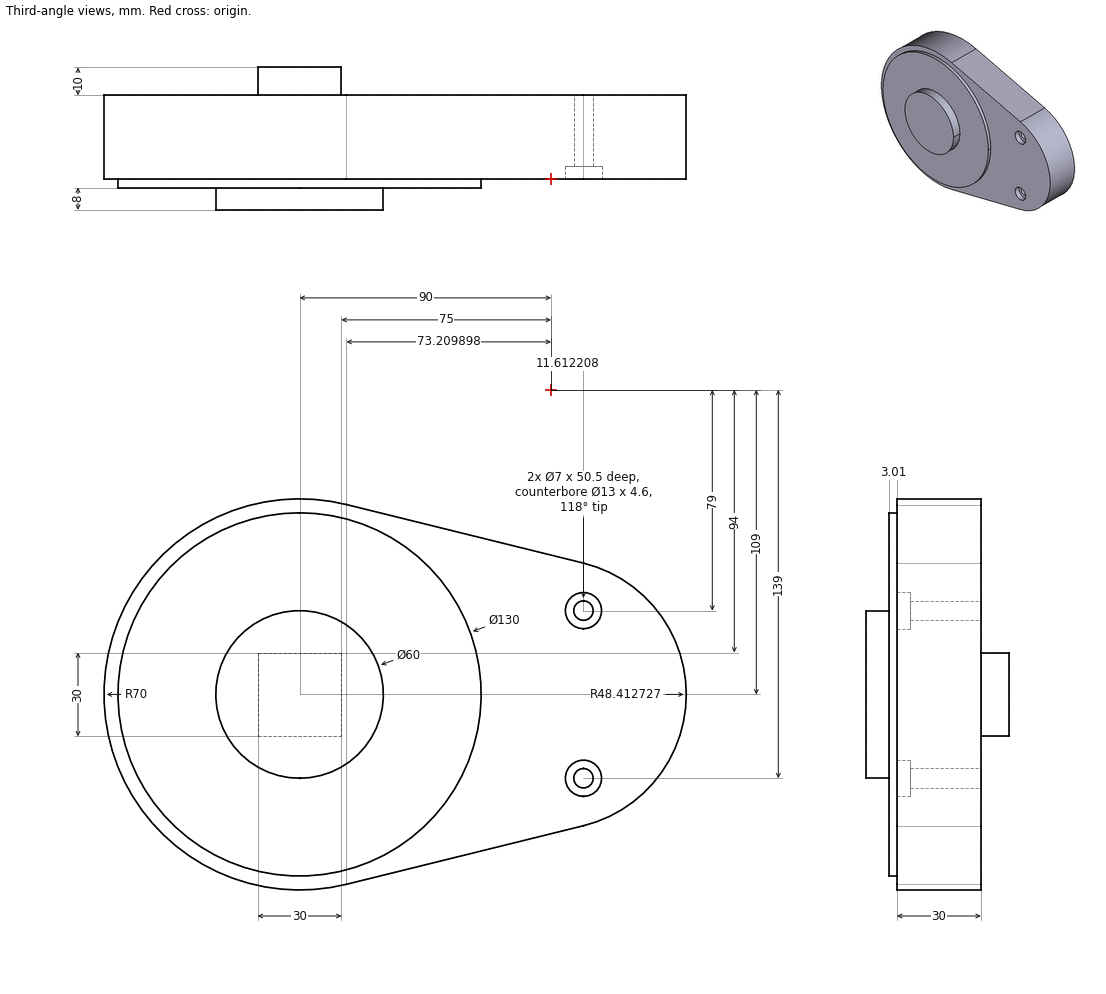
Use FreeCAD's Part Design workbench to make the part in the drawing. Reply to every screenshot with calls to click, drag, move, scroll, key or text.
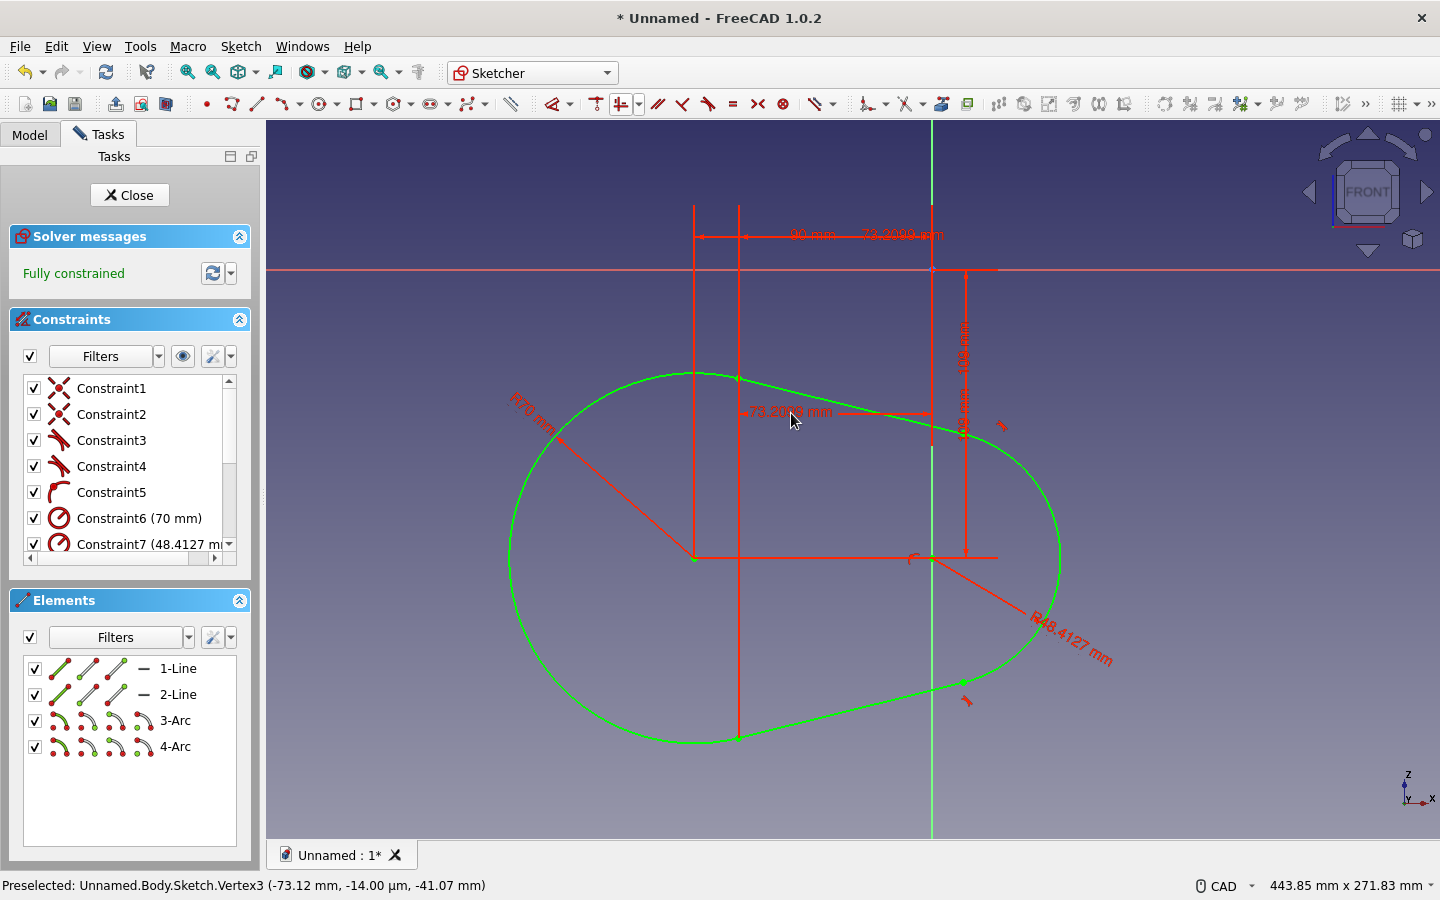
click(130, 195)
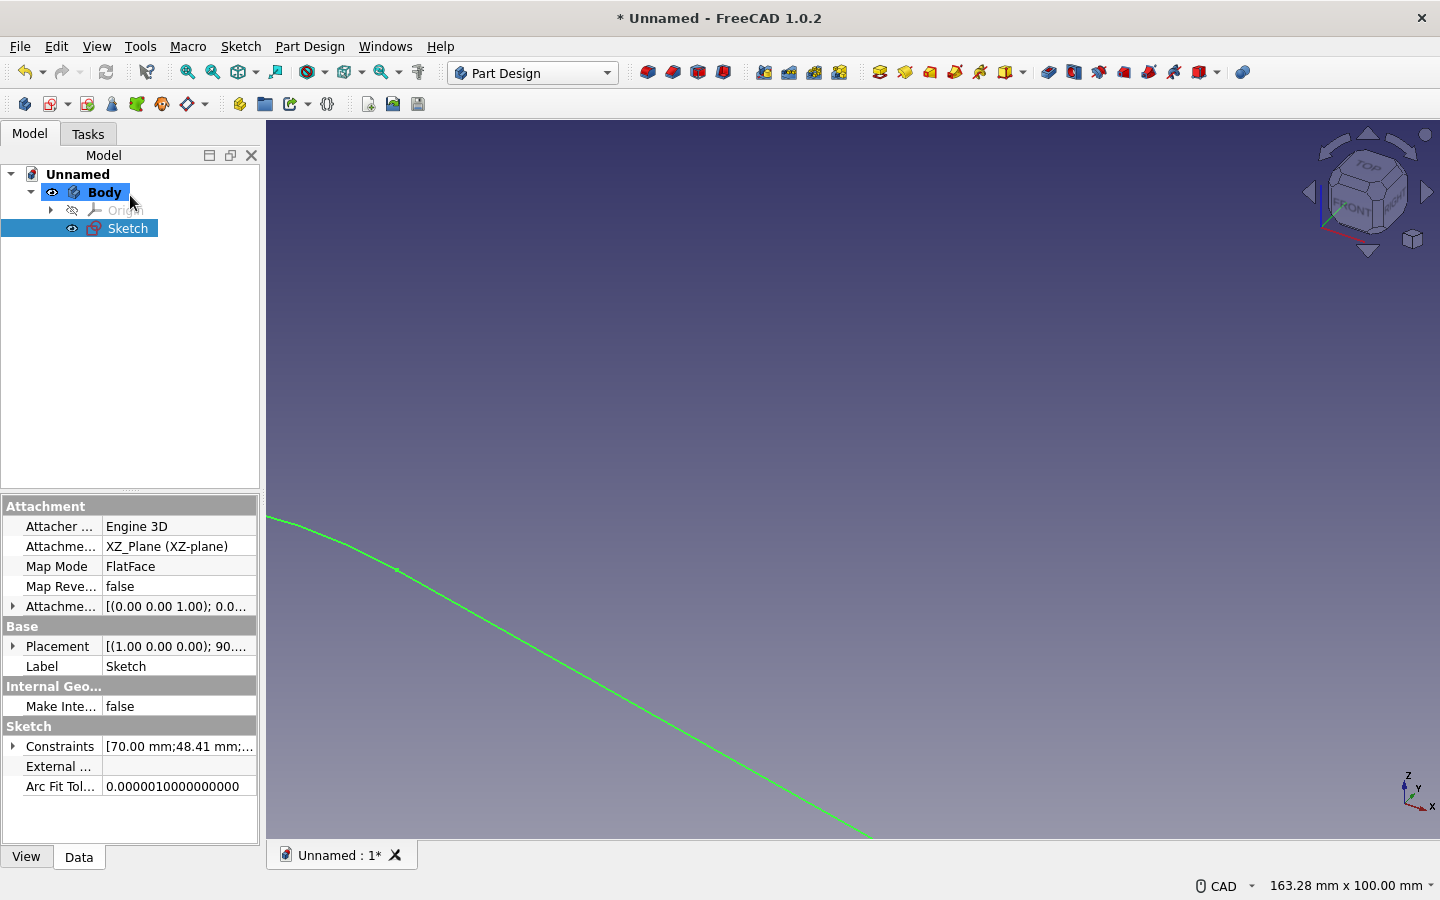
click(880, 72)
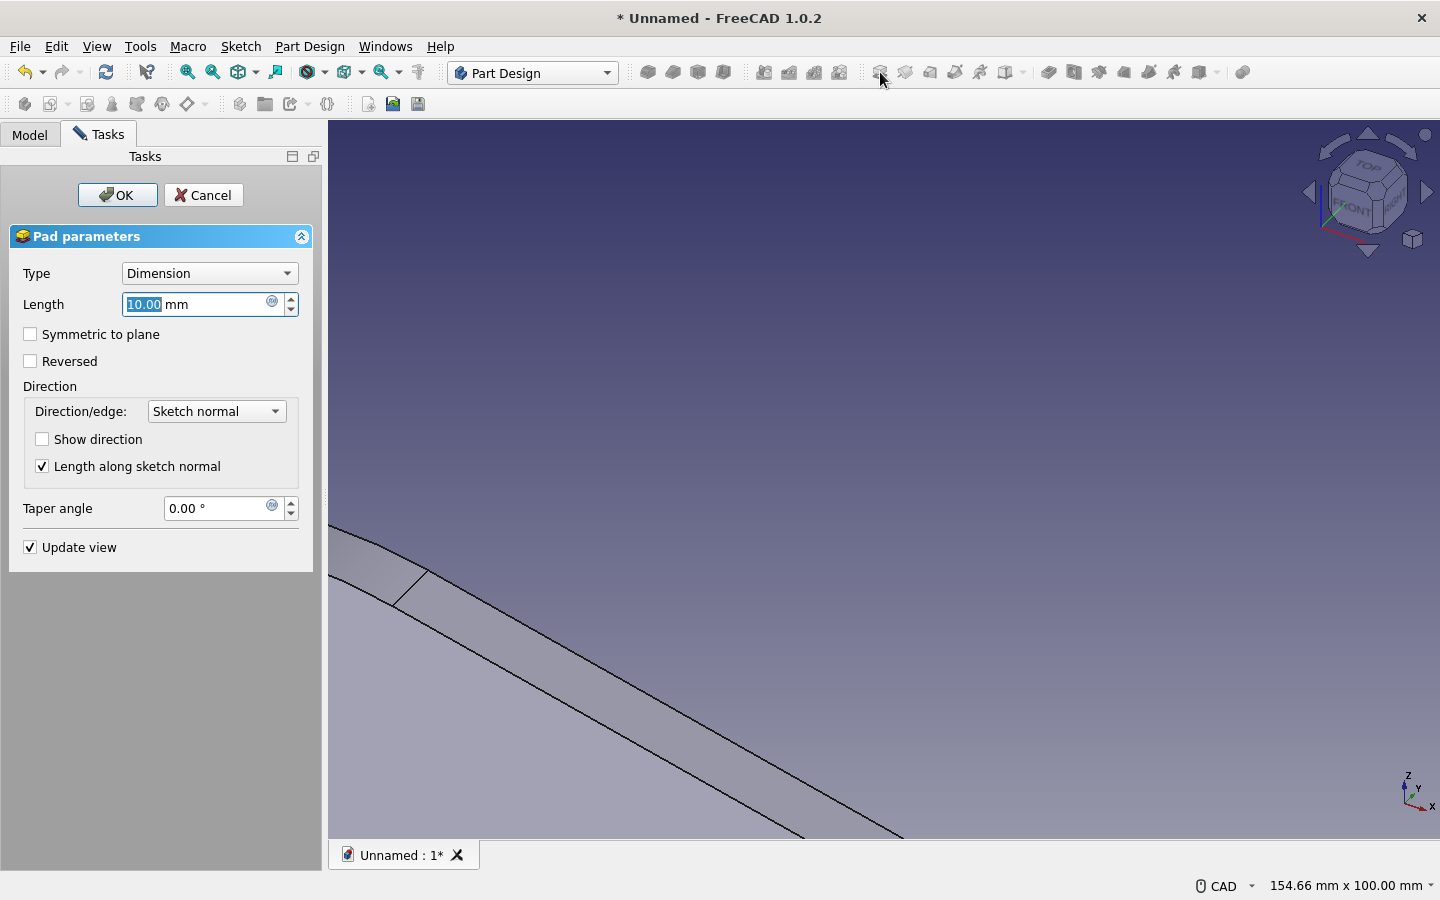
text(30)
key(Tab)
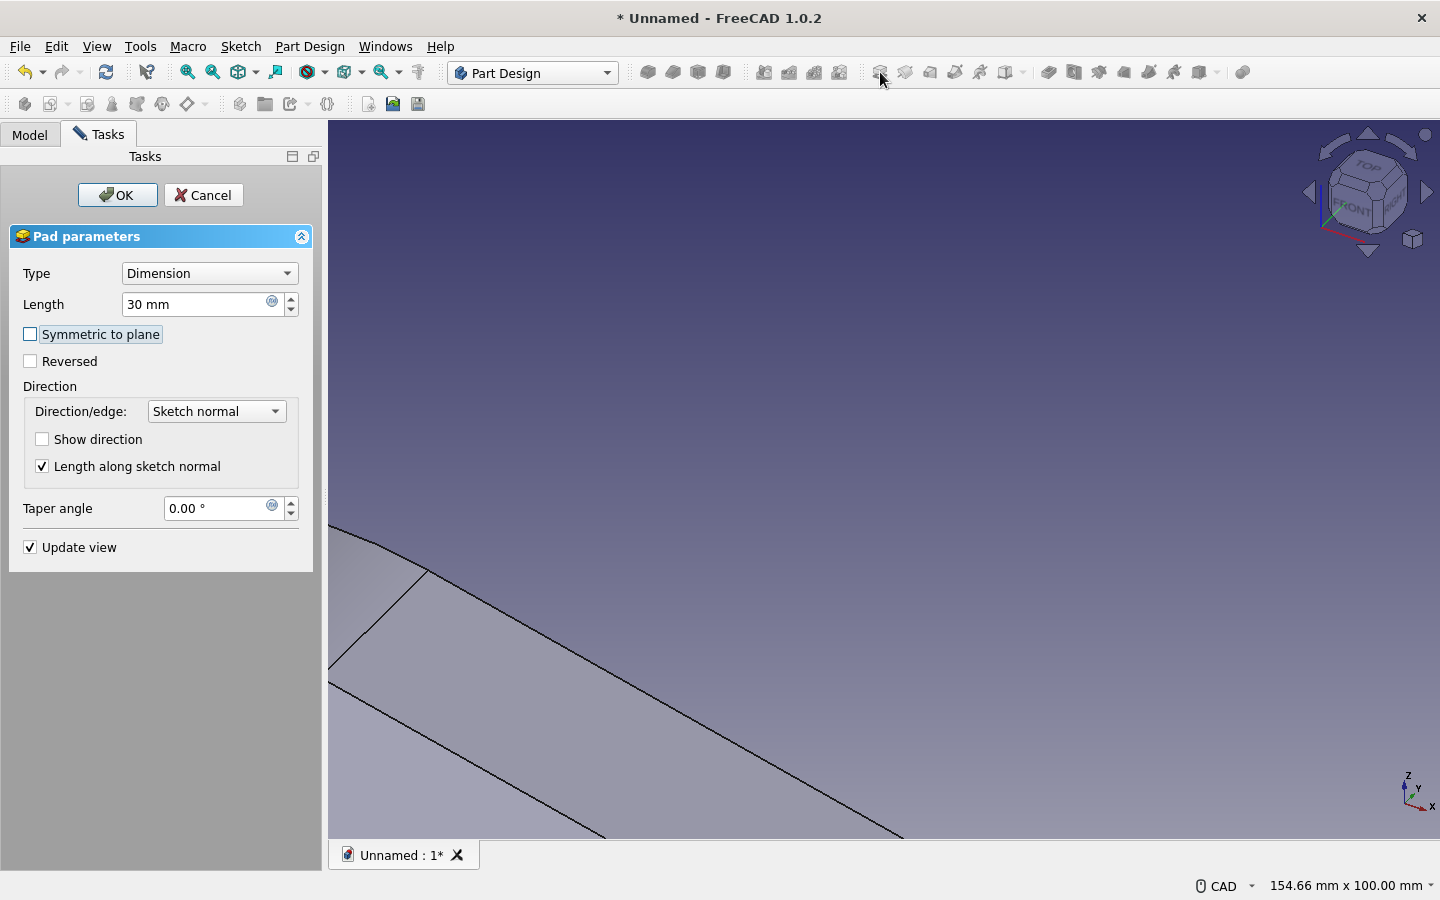
click(31, 361)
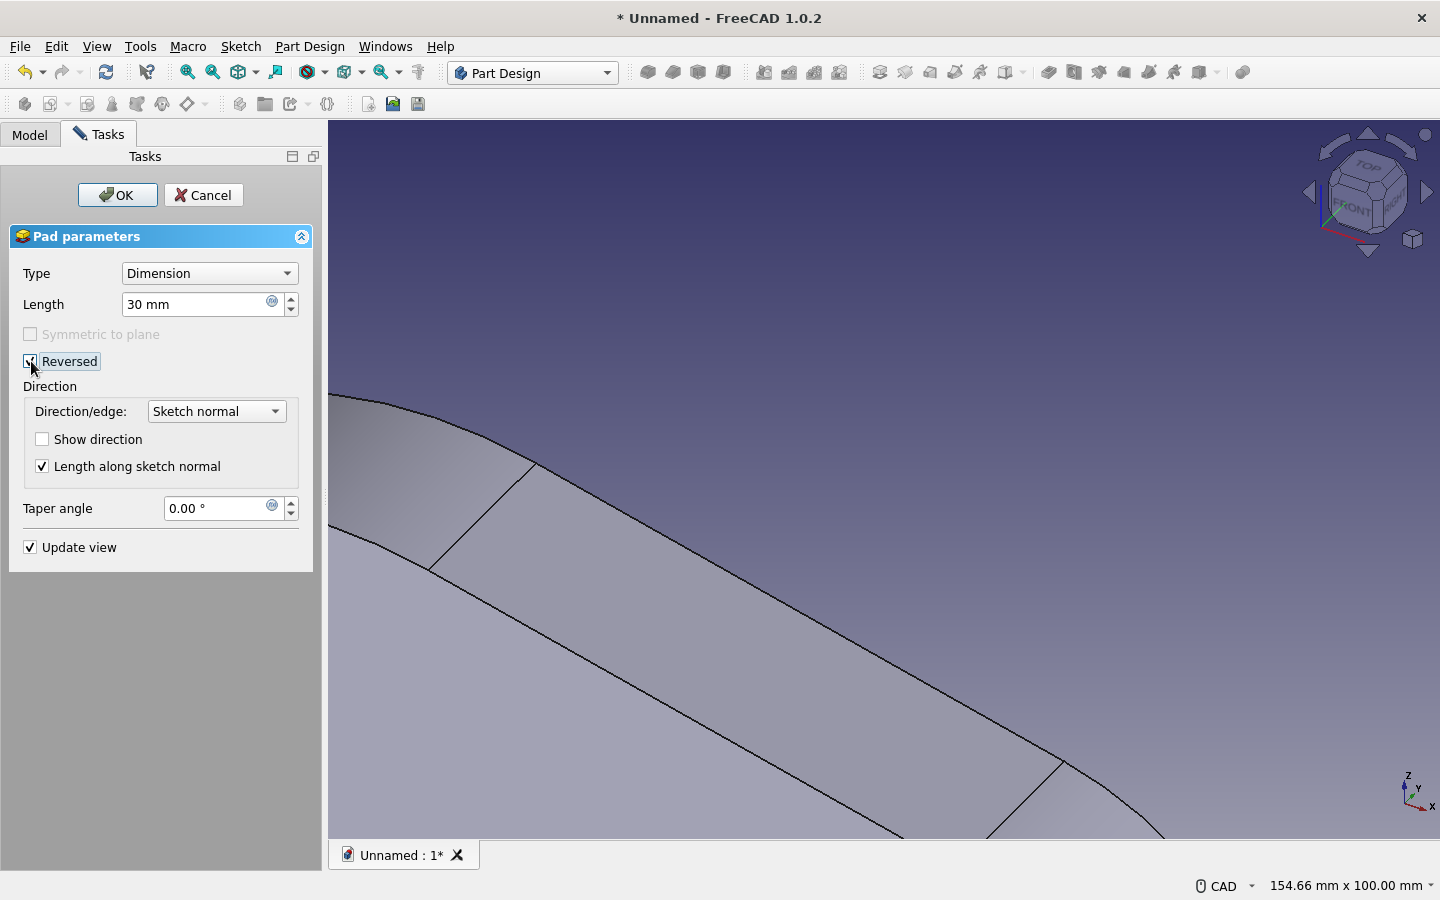
click(118, 195)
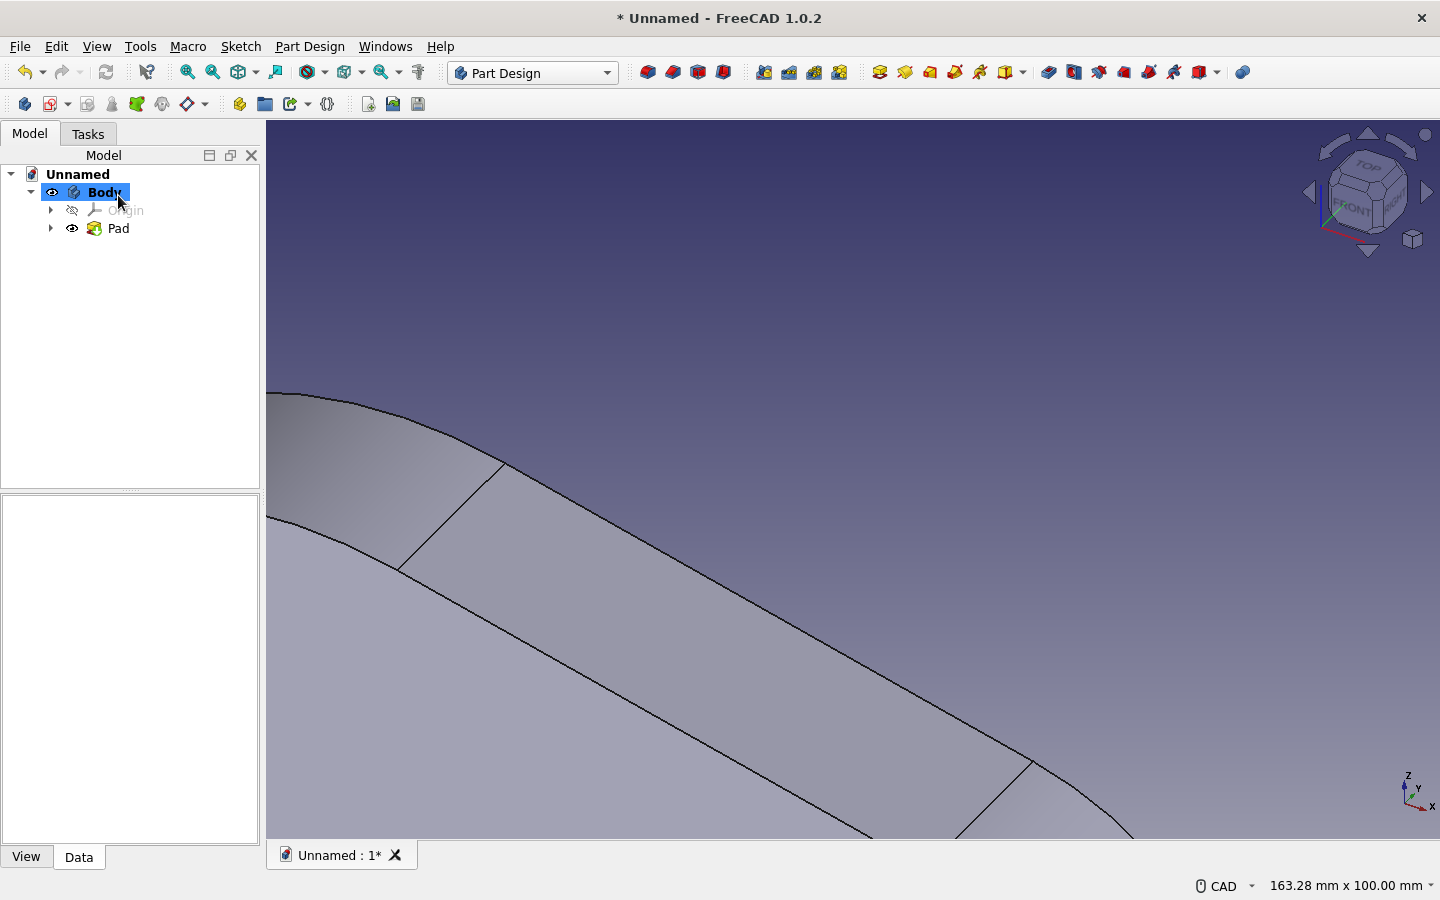
key(v)
key(f)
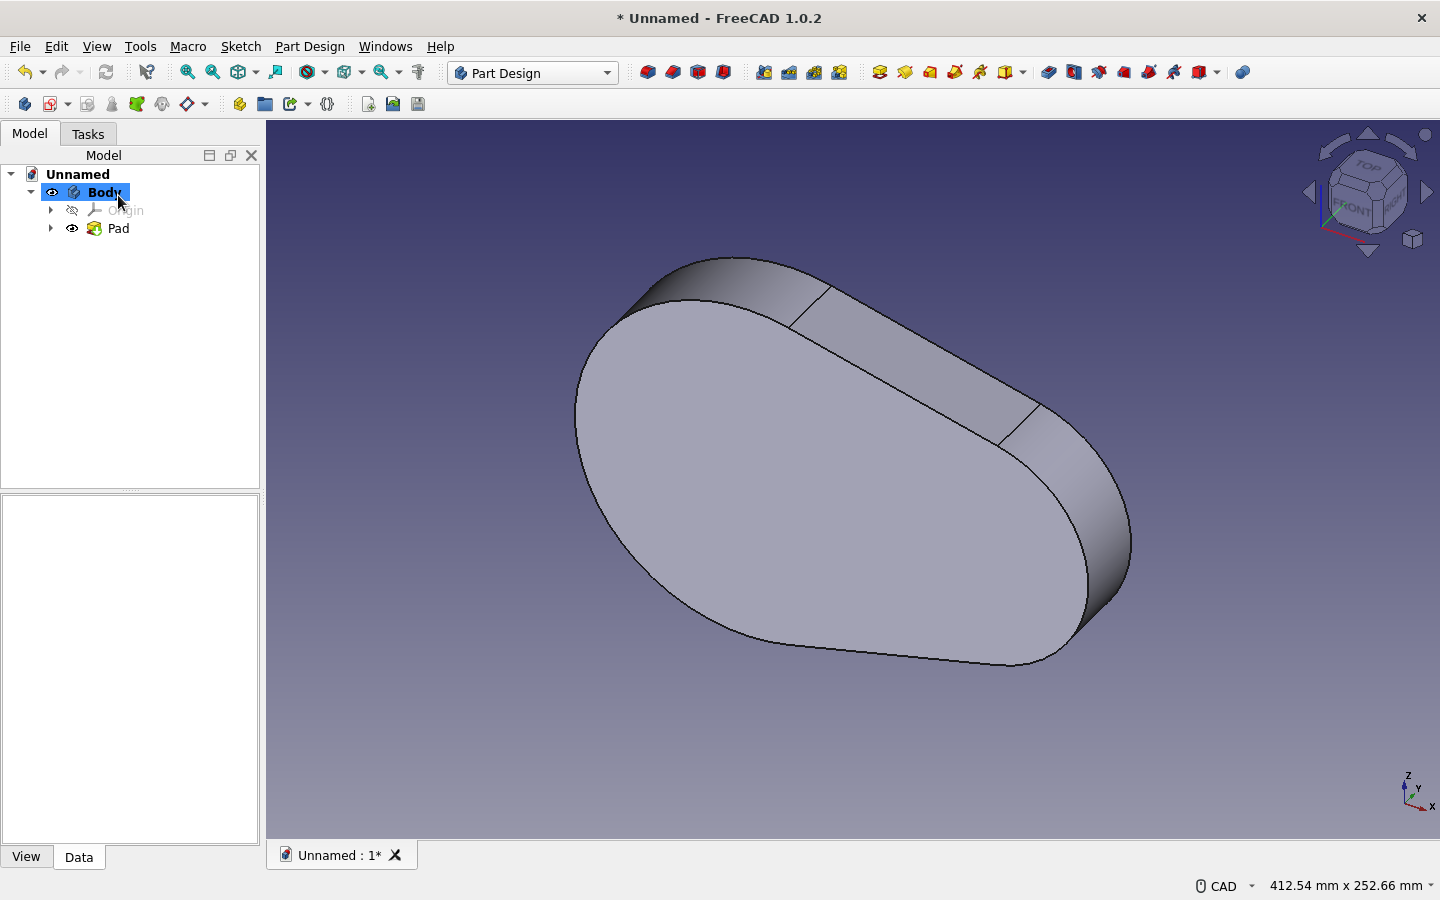
key(4)